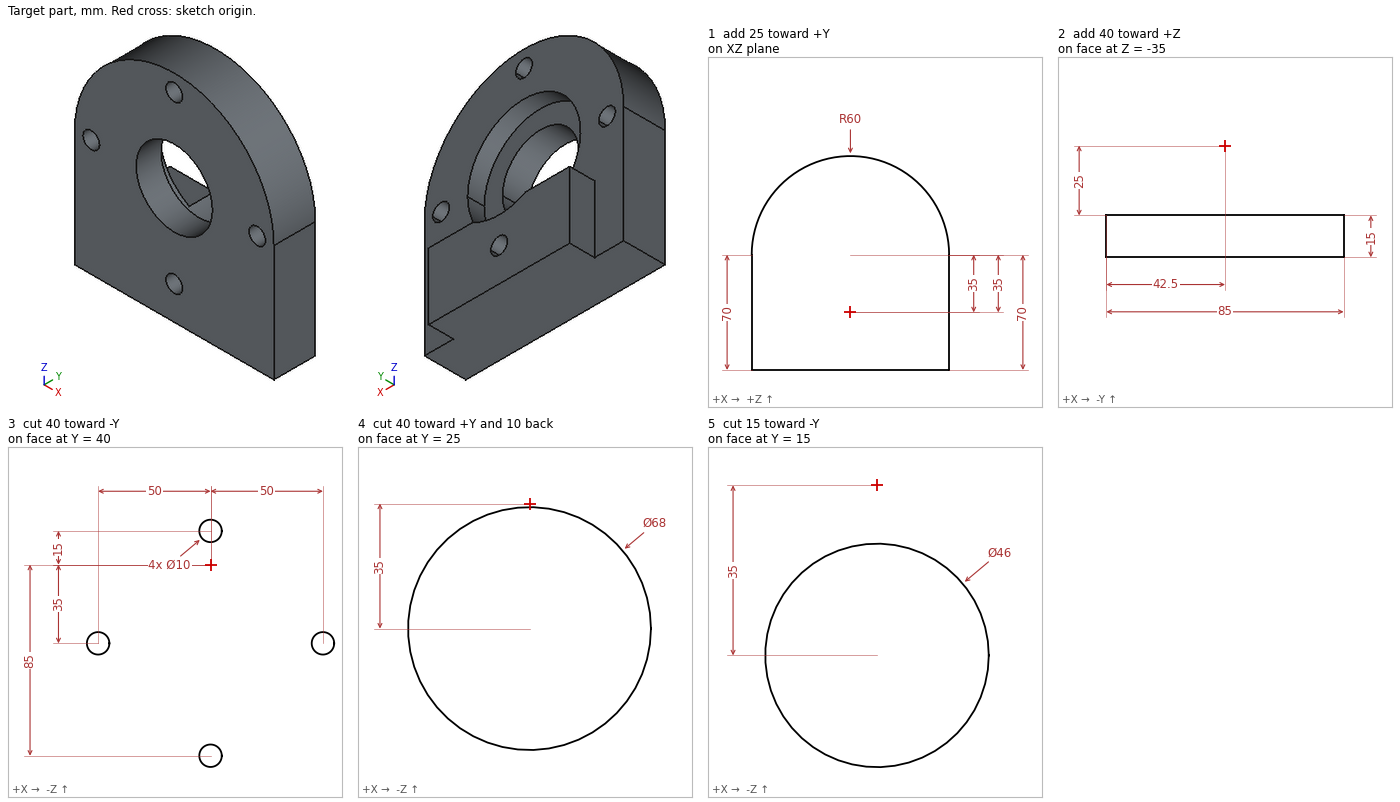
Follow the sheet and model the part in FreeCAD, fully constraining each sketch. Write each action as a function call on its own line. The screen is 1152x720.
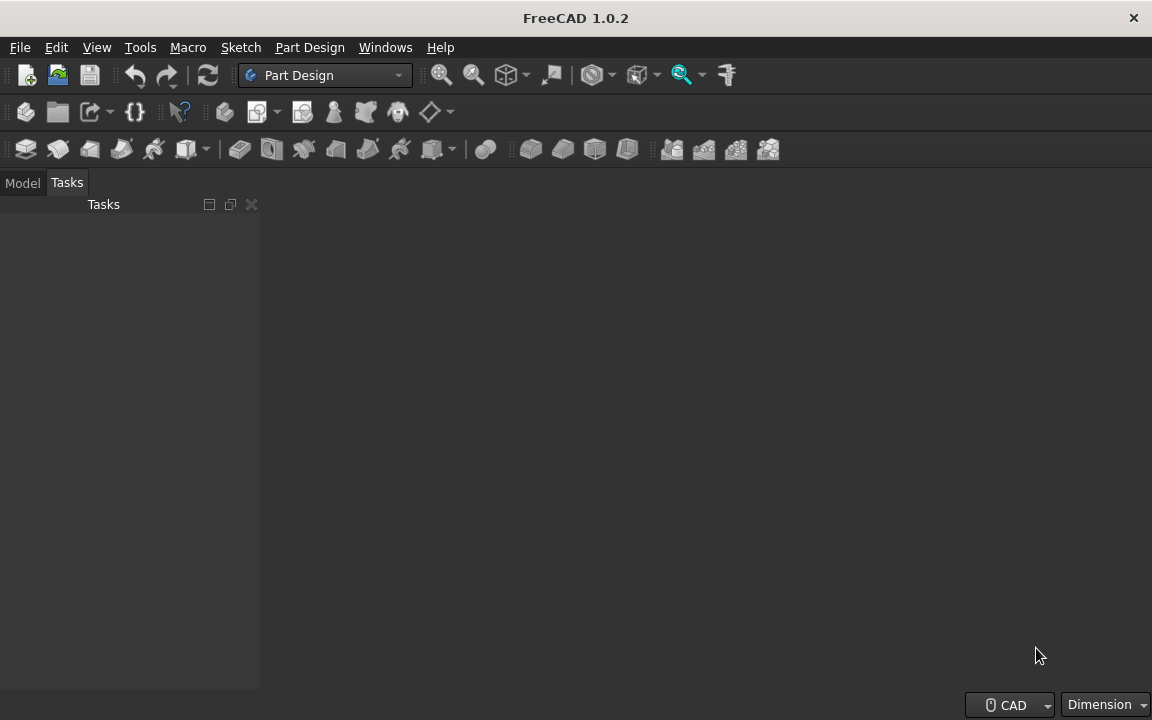
click(26, 76)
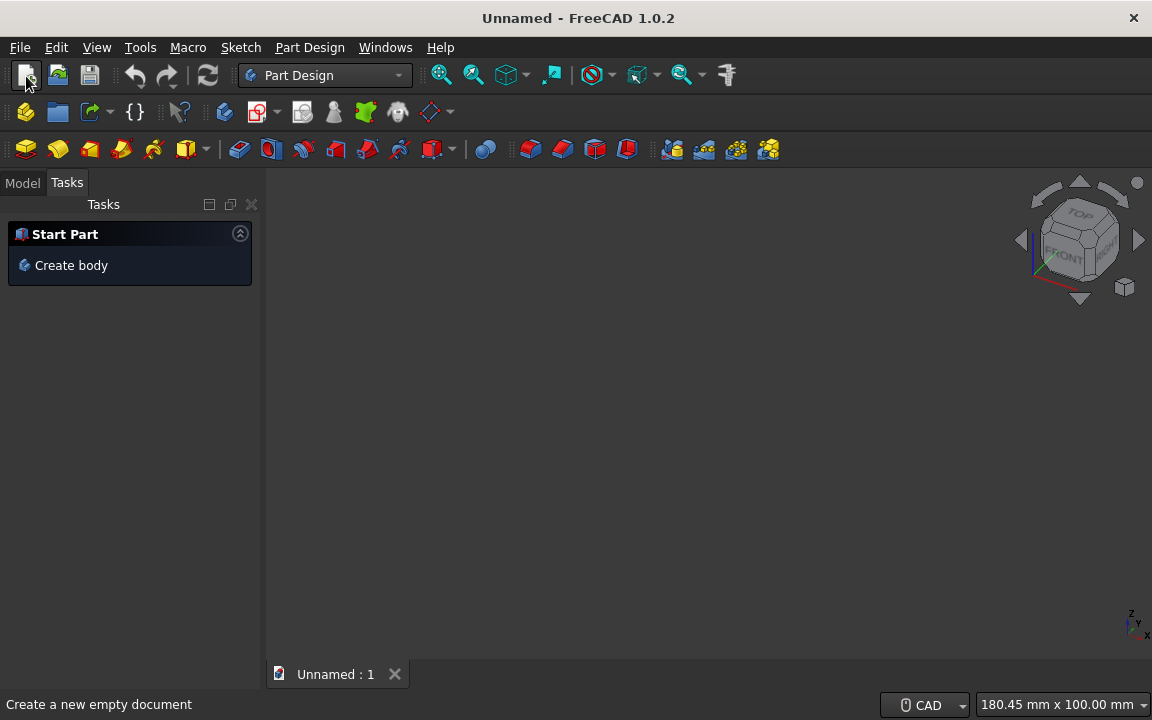
click(258, 112)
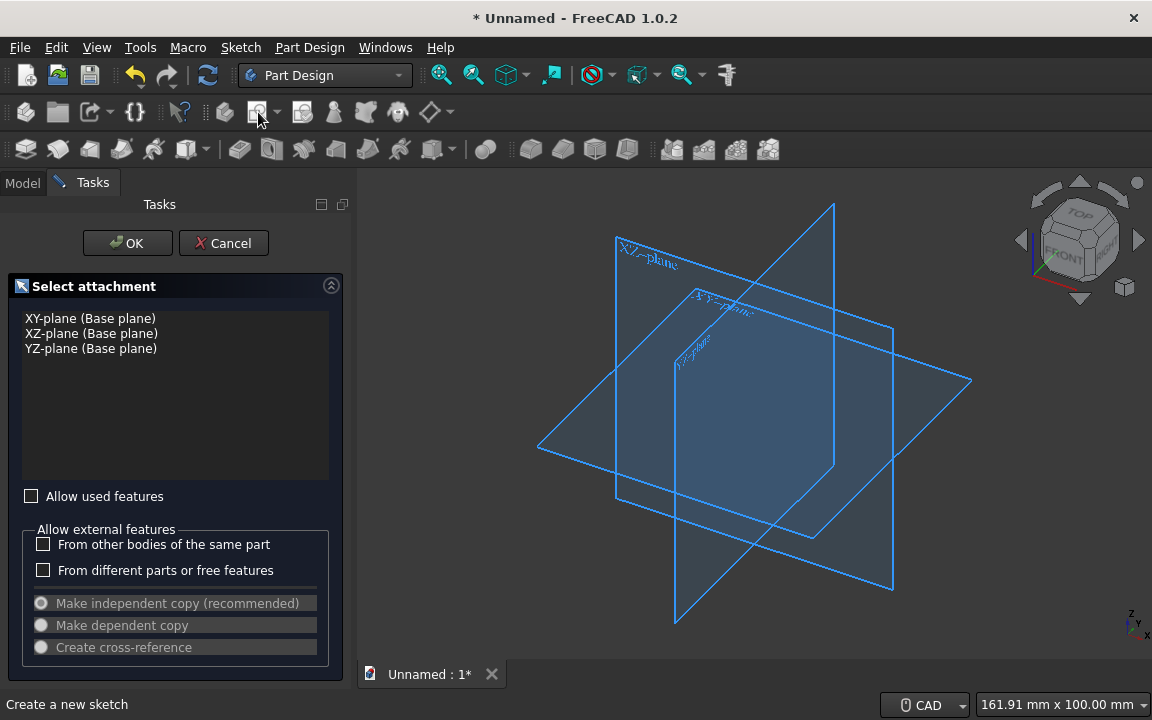
click(82, 334)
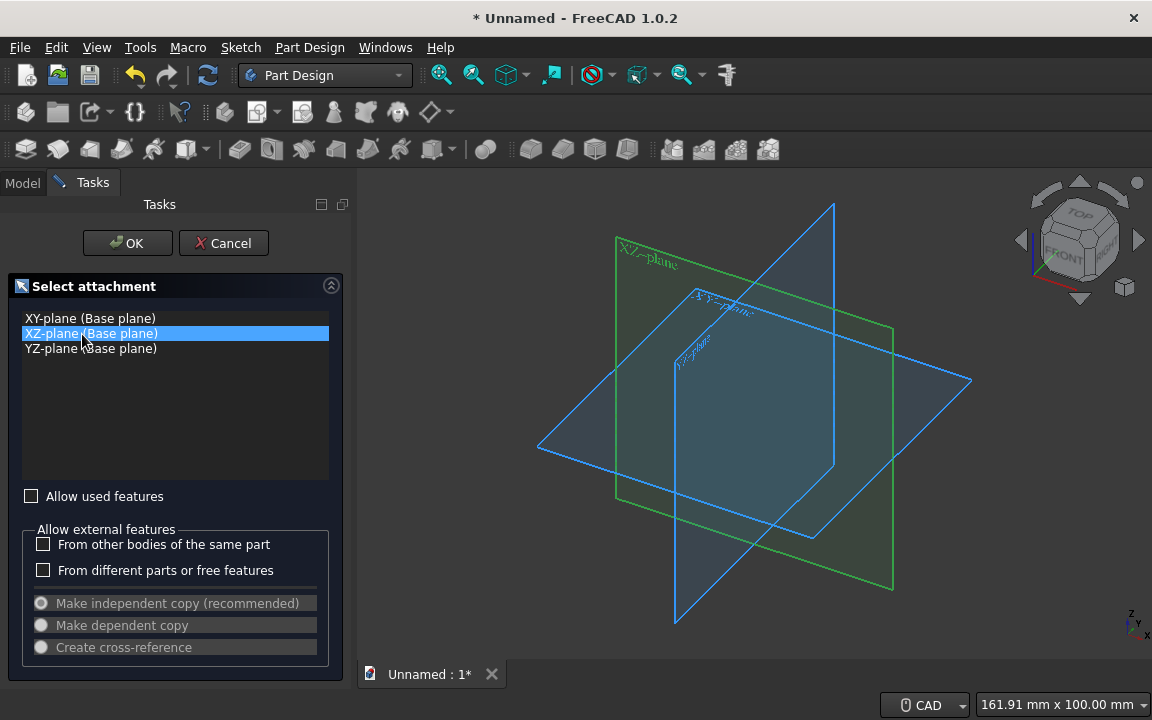
click(128, 243)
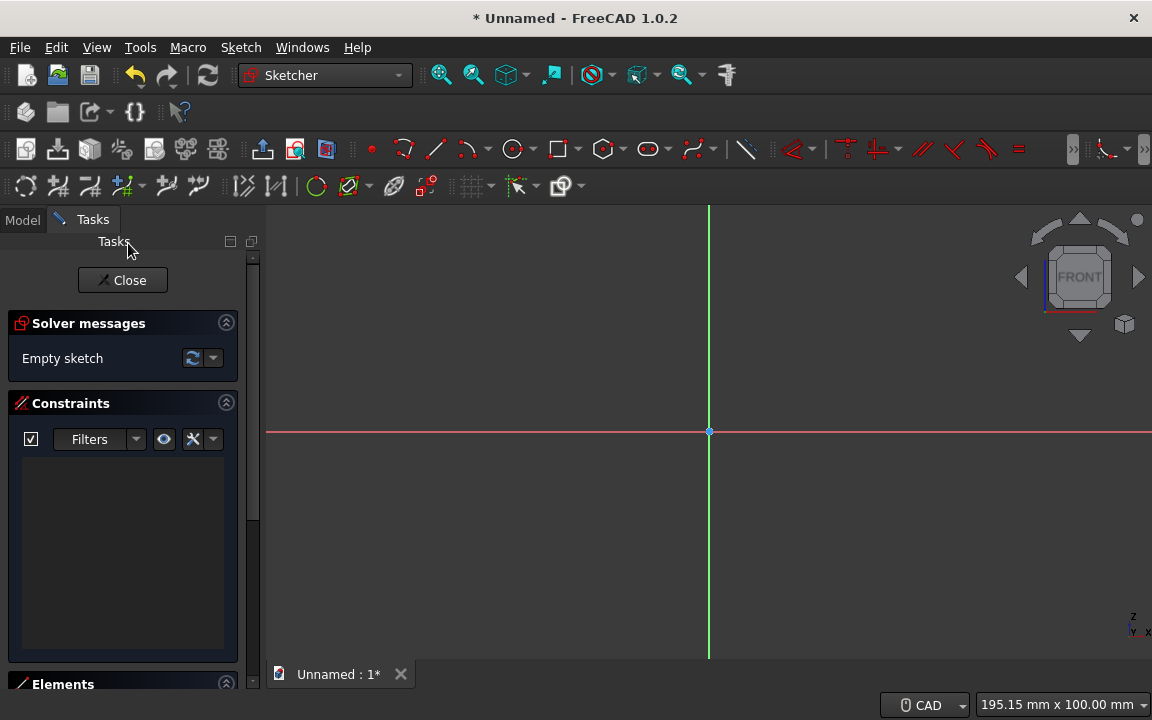
scroll(585, 543, down, 4)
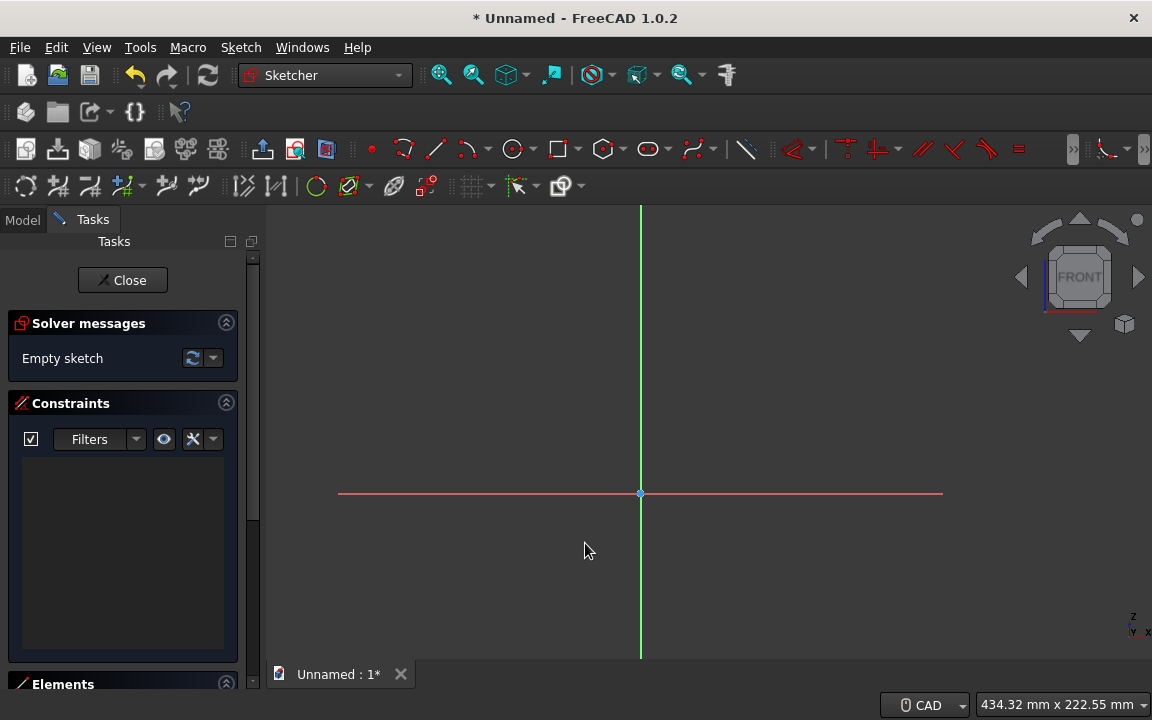
key(g)
key(m)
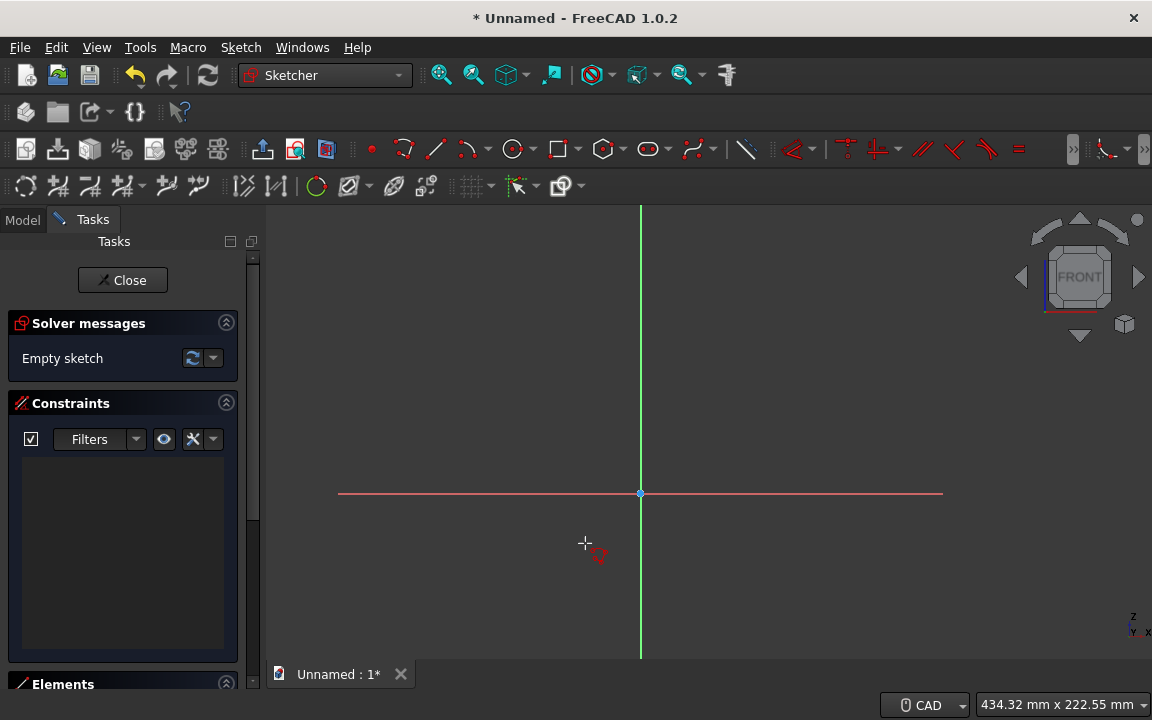
click(763, 422)
click(763, 565)
click(519, 565)
click(519, 422)
right_click(519, 422)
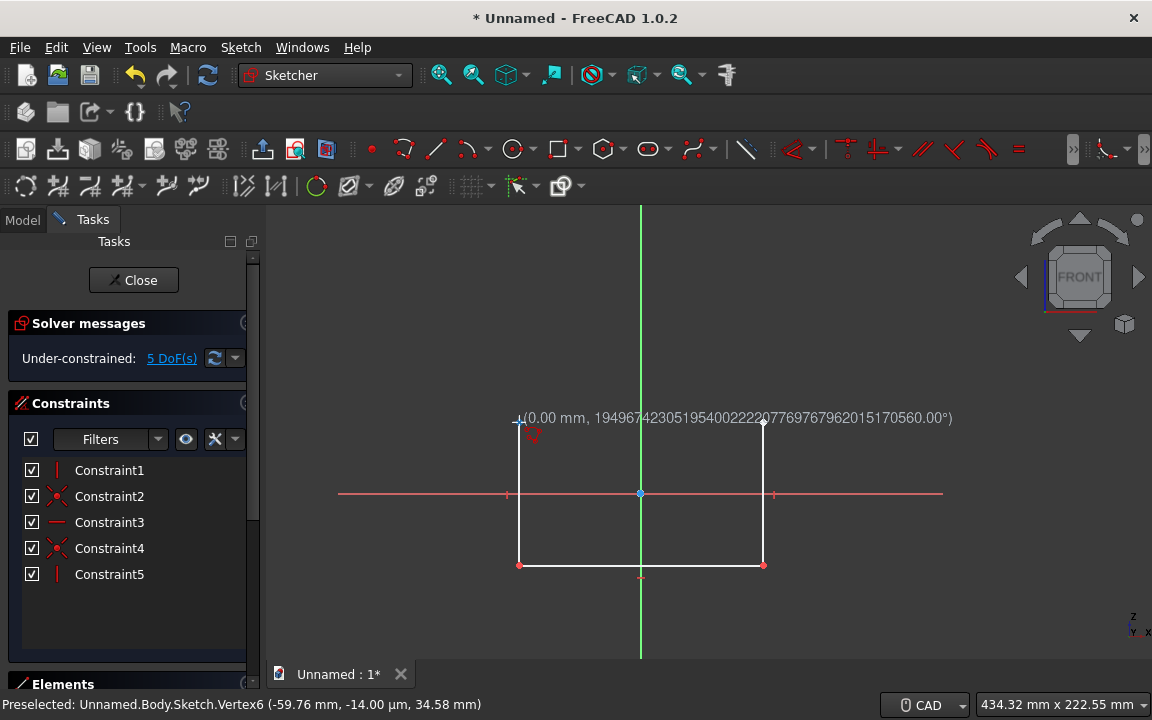
key(g)
key(3)
key(a)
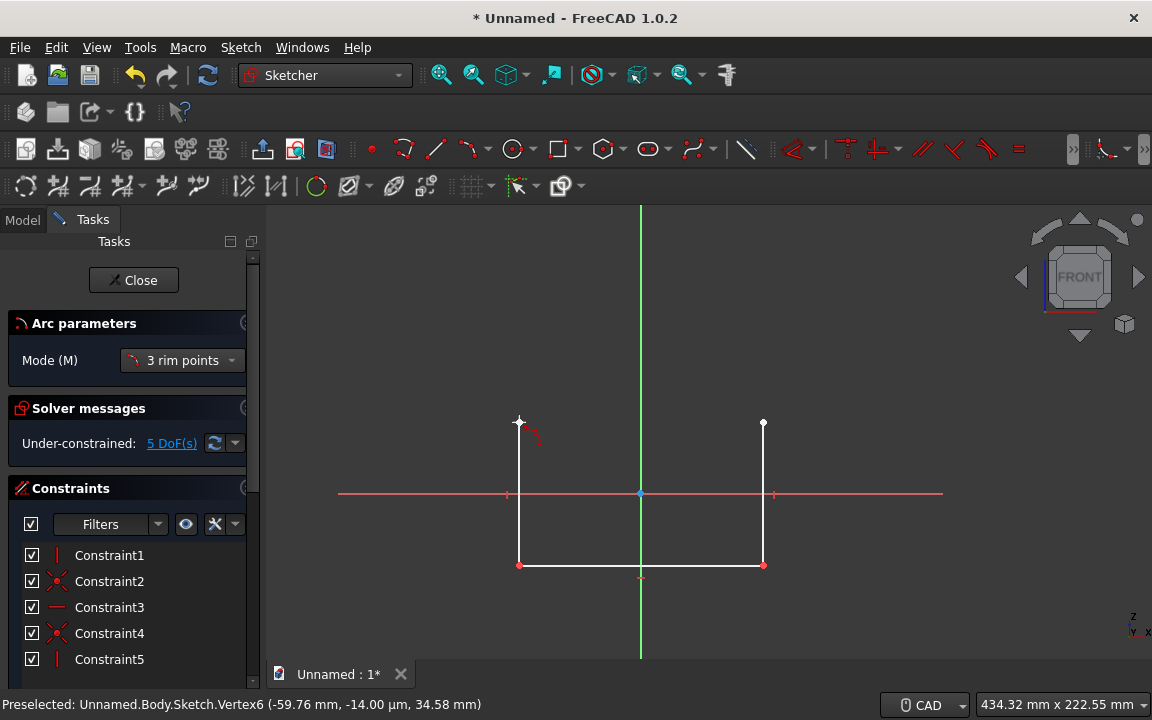
click(519, 423)
click(763, 423)
click(679, 306)
key(Escape)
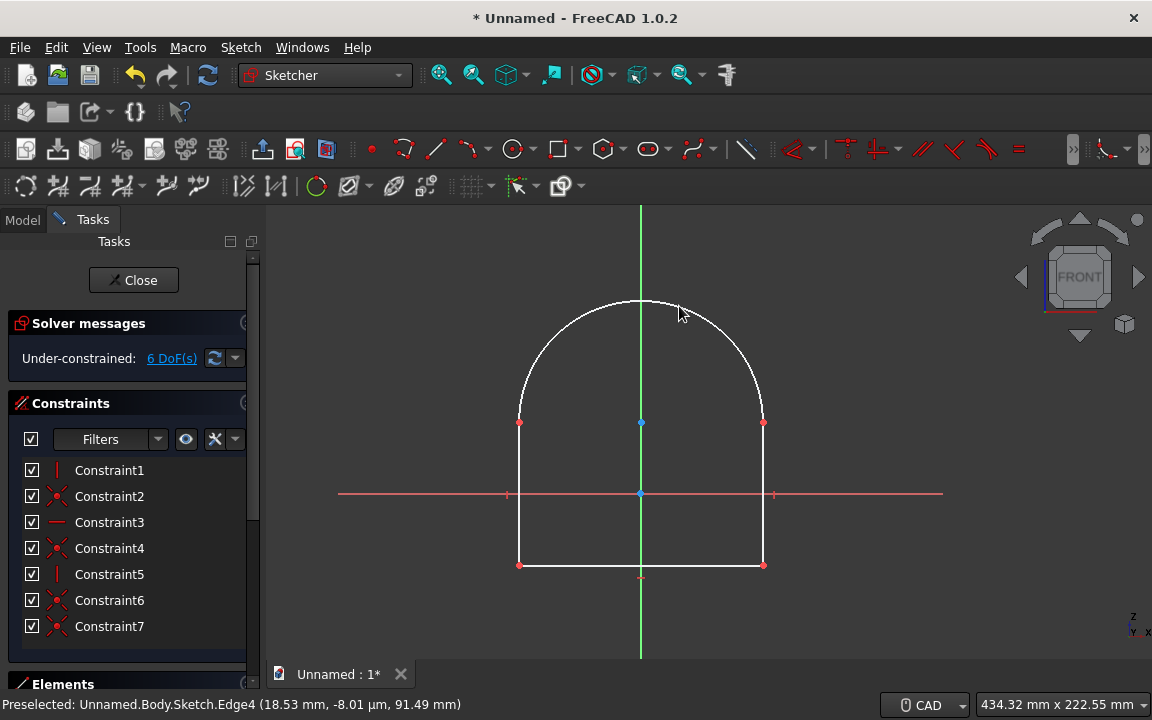
click(641, 423)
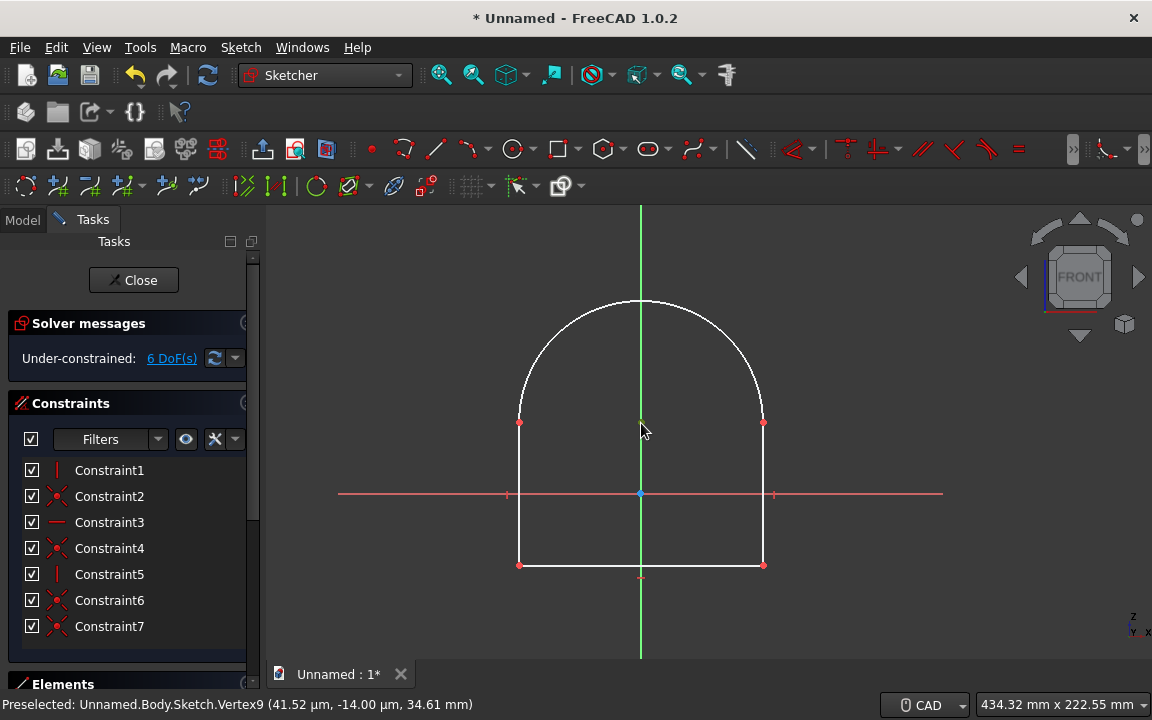
click(641, 603)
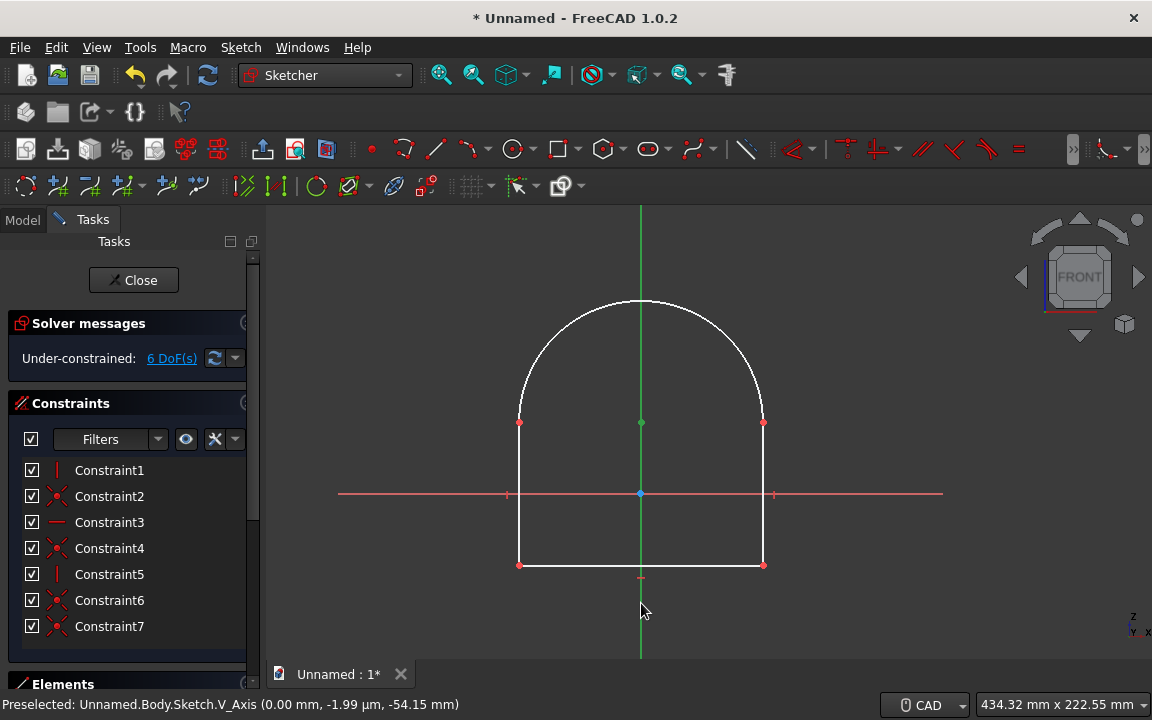
key(c)